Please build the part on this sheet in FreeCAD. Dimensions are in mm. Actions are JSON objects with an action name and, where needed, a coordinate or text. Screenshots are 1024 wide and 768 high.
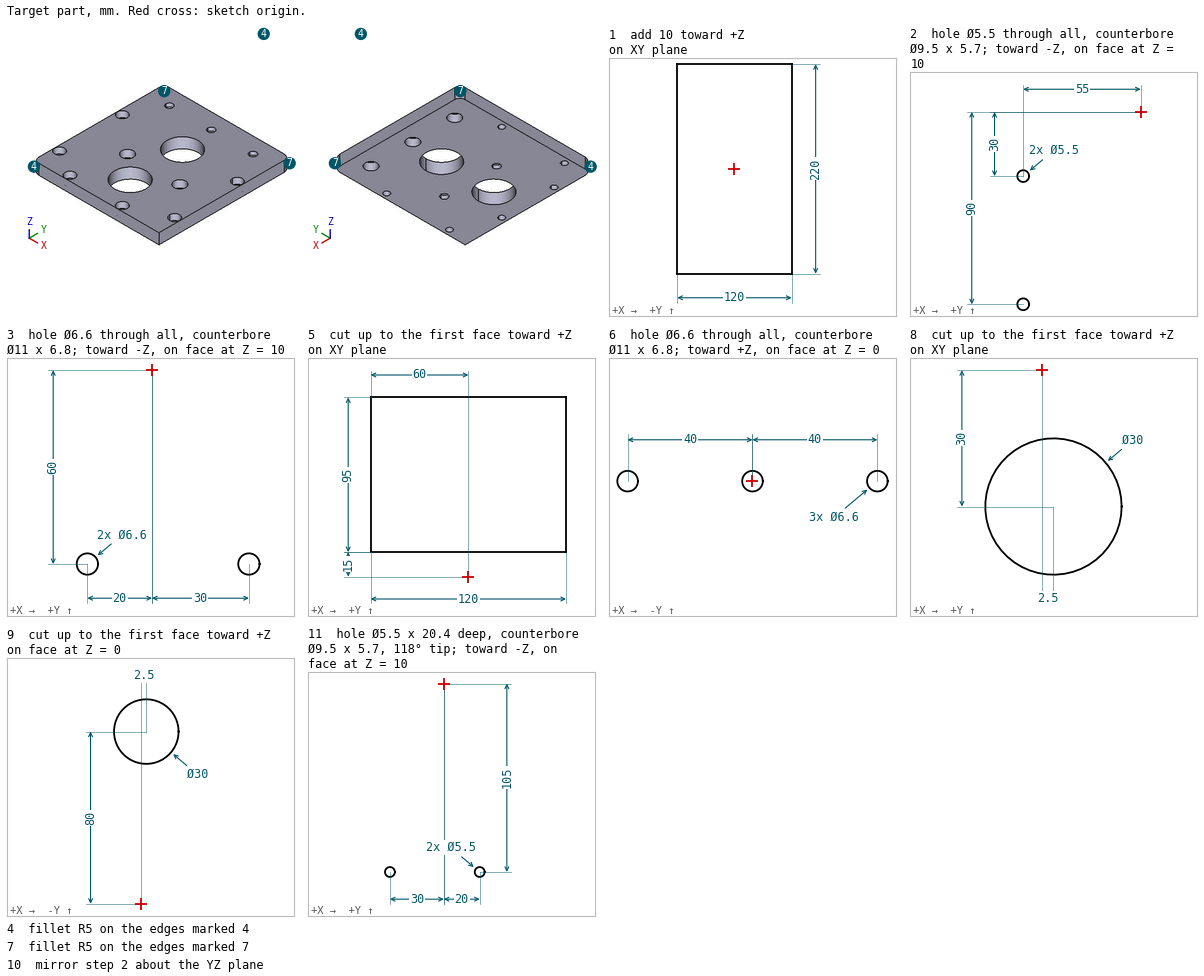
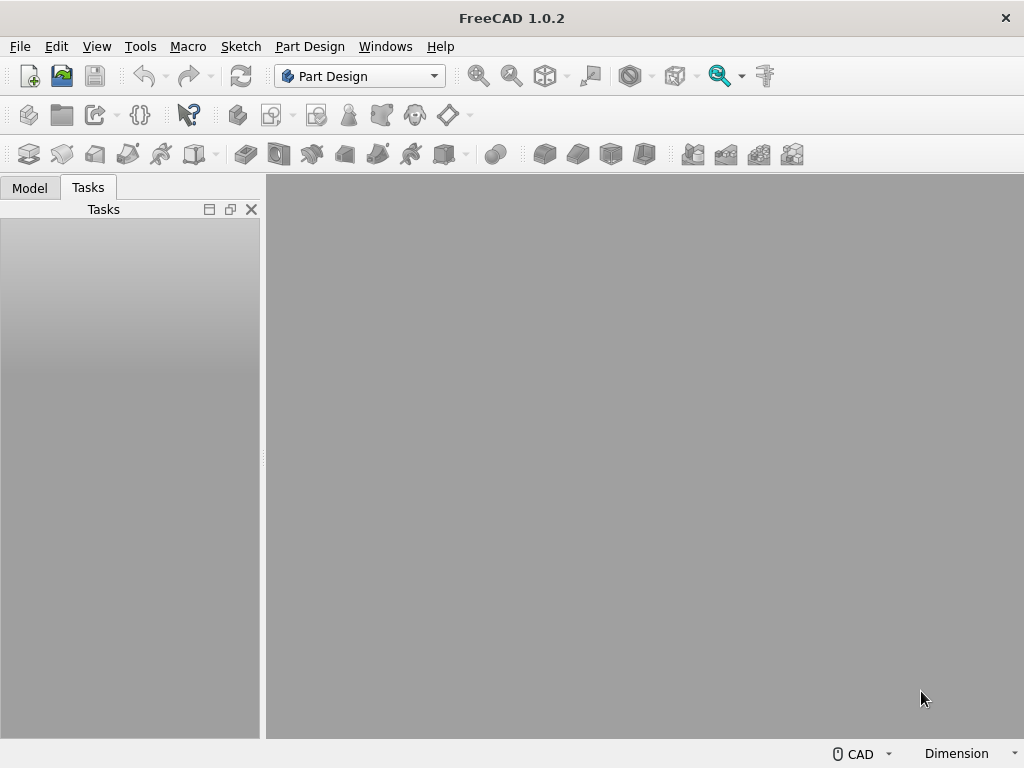
{"action": "left_click", "coordinate": [29, 76]}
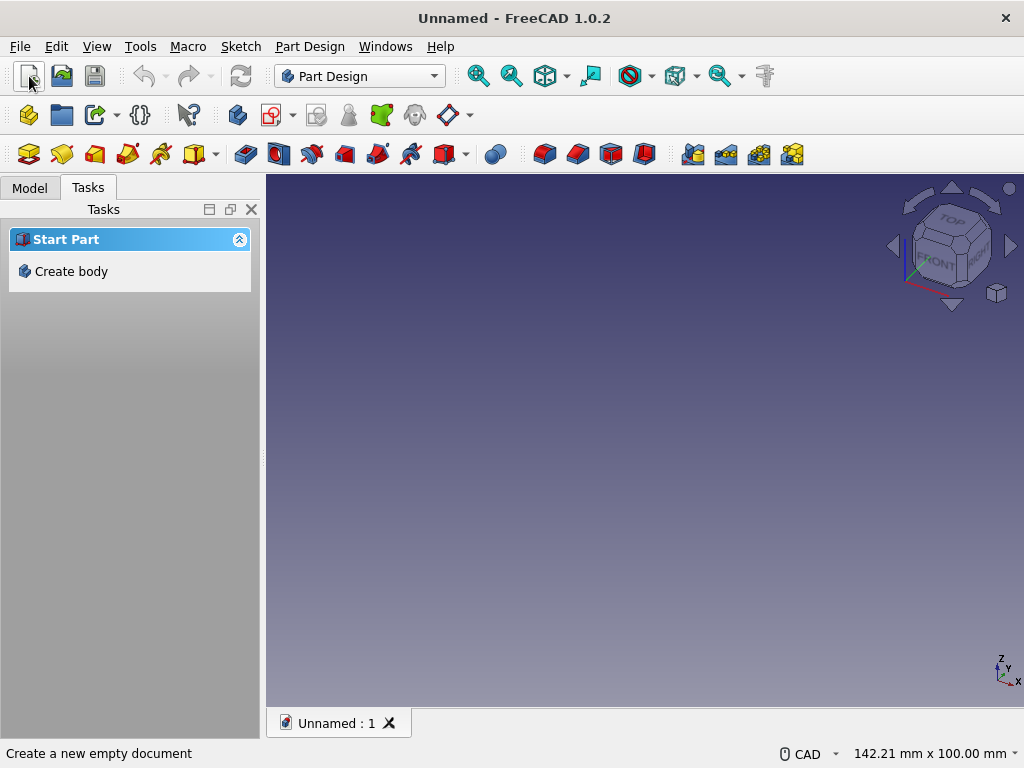
{"action": "left_click", "coordinate": [270, 116]}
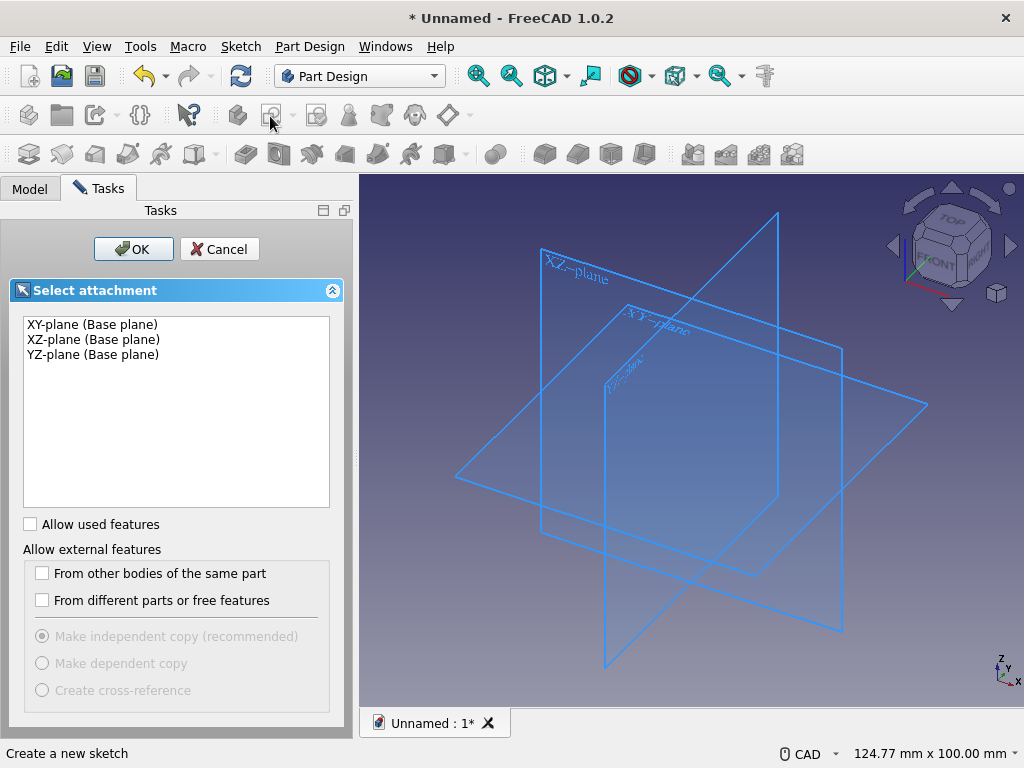
{"action": "left_click", "coordinate": [84, 324]}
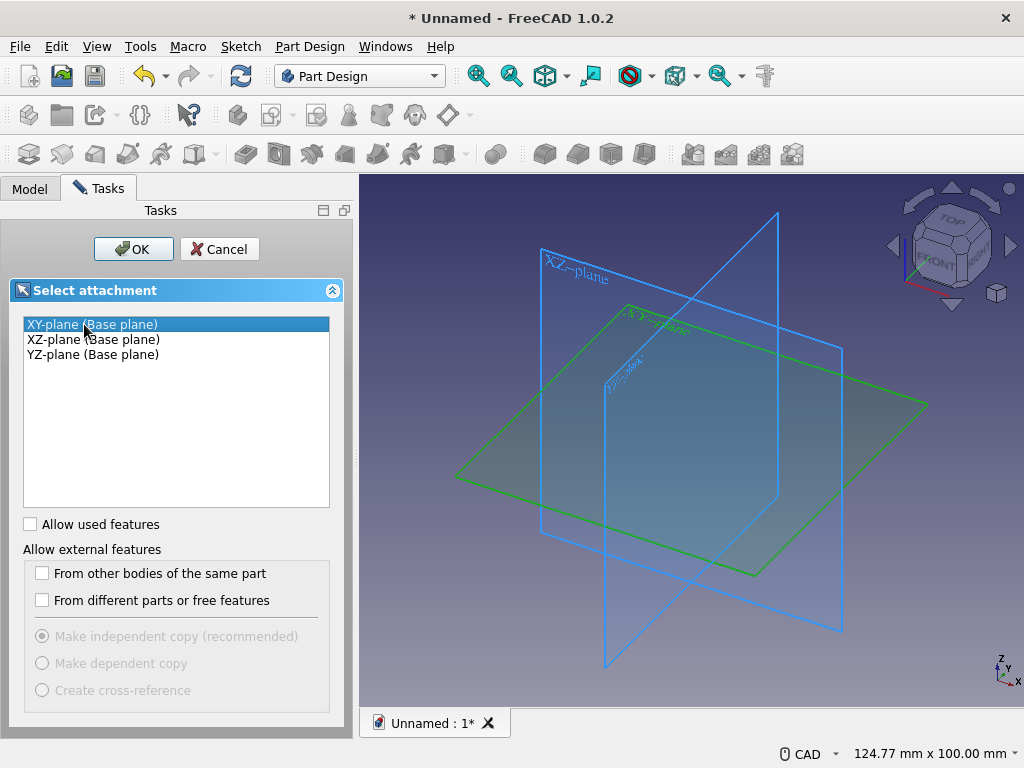
{"action": "left_click", "coordinate": [134, 249]}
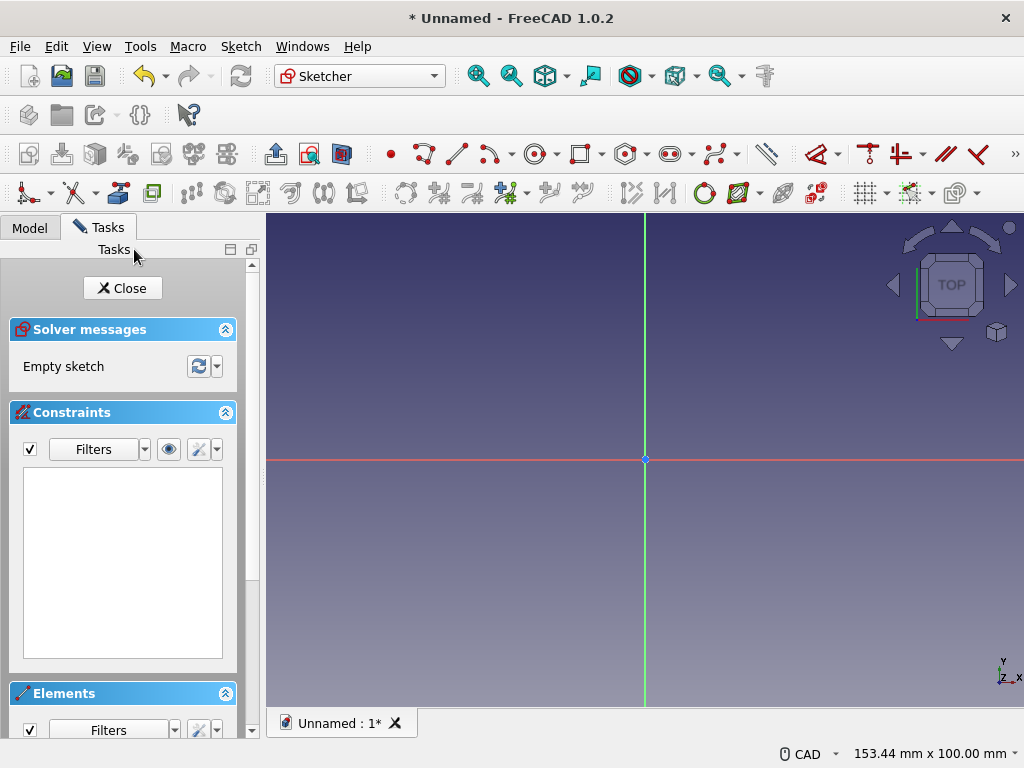
{"action": "scroll", "coordinate": [547, 460], "scroll_direction": "down", "scroll_amount": 6}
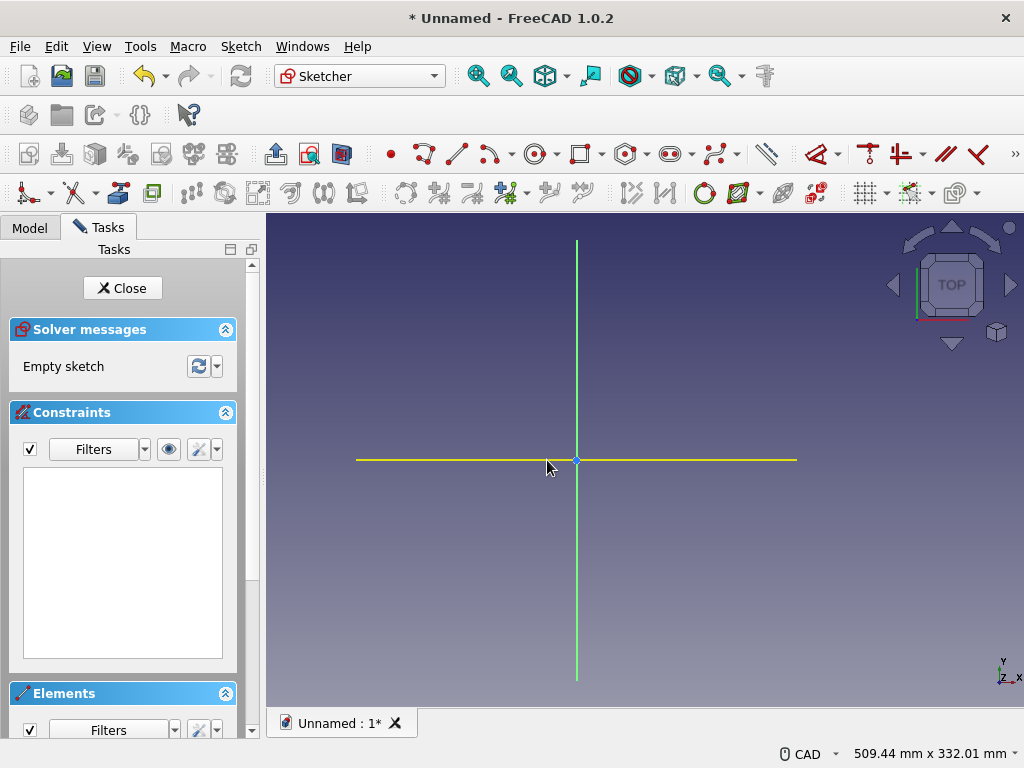
{"action": "left_click", "coordinate": [602, 154]}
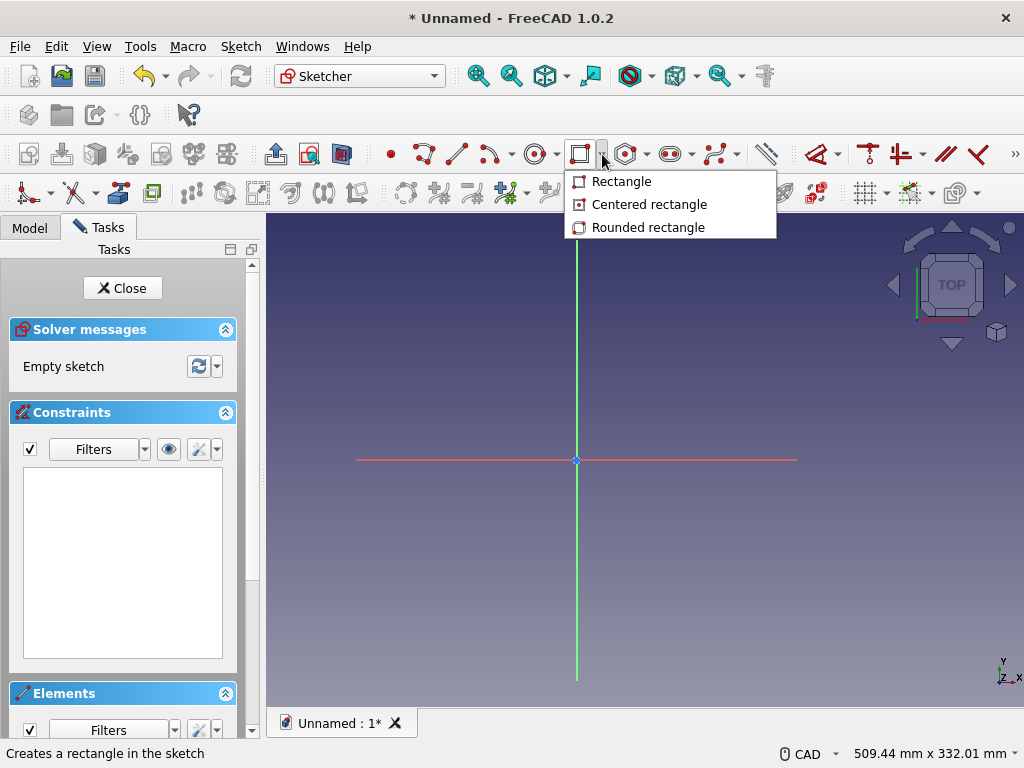
{"action": "left_click", "coordinate": [670, 204]}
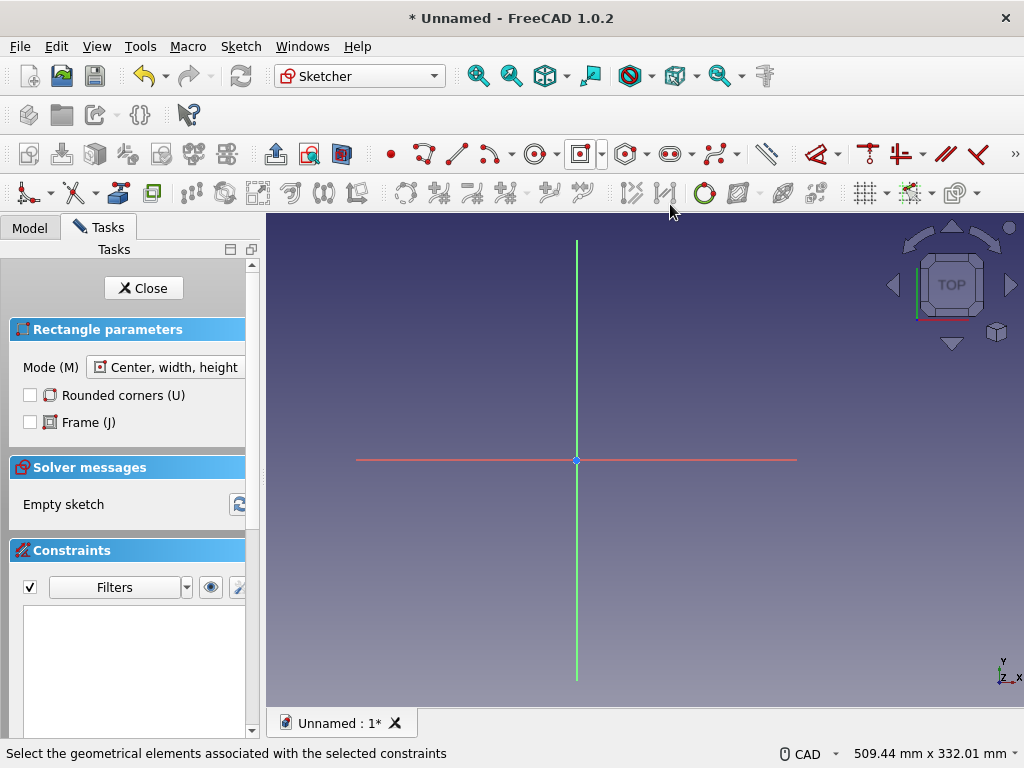
{"action": "left_click", "coordinate": [577, 460]}
{"action": "left_click", "coordinate": [666, 297]}
{"action": "key", "text": "Escape"}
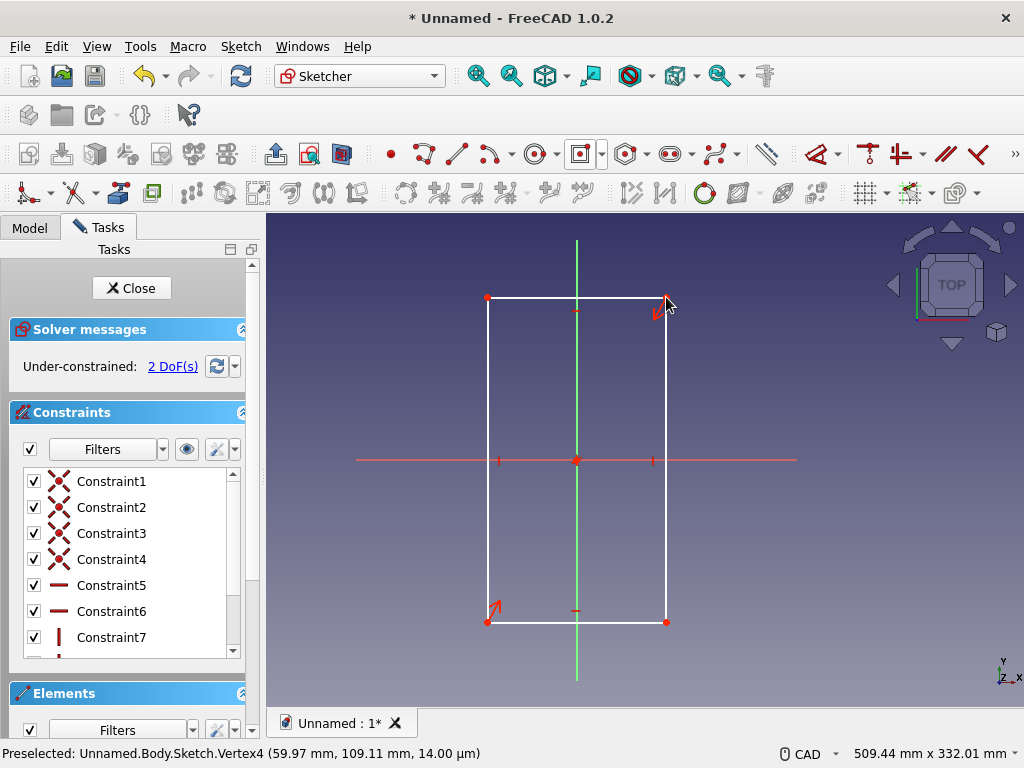
{"action": "left_click", "coordinate": [816, 154]}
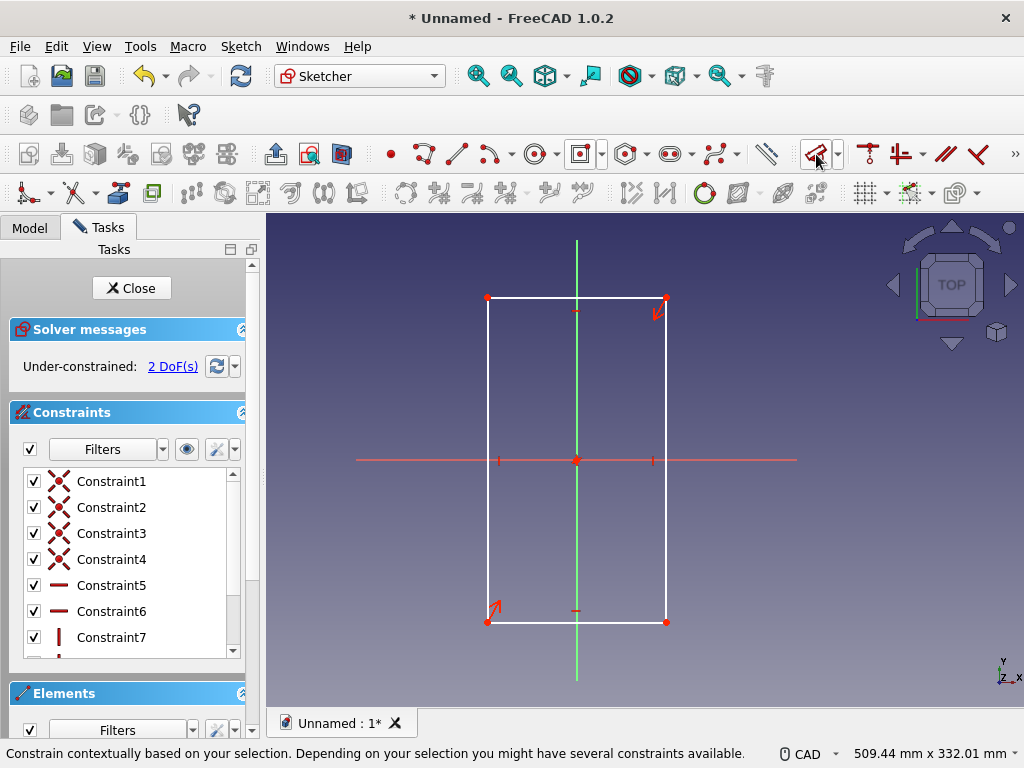
{"action": "left_click", "coordinate": [541, 623]}
{"action": "left_click", "coordinate": [536, 657]}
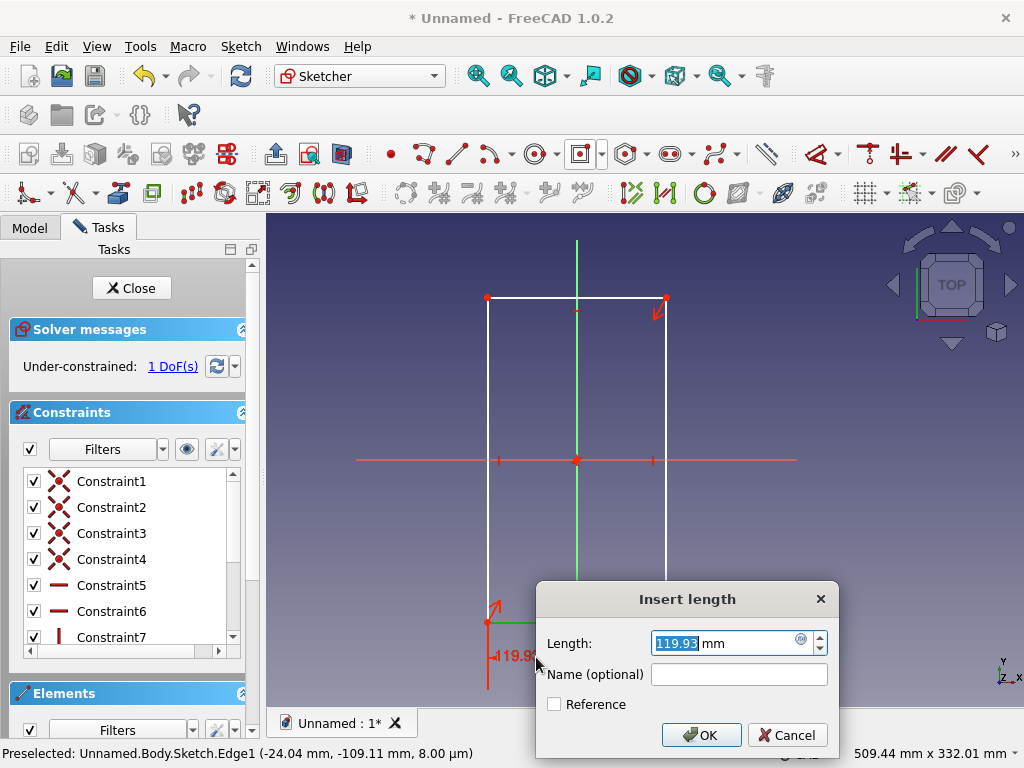
{"action": "type", "text": "120"}
{"action": "key", "text": "Return"}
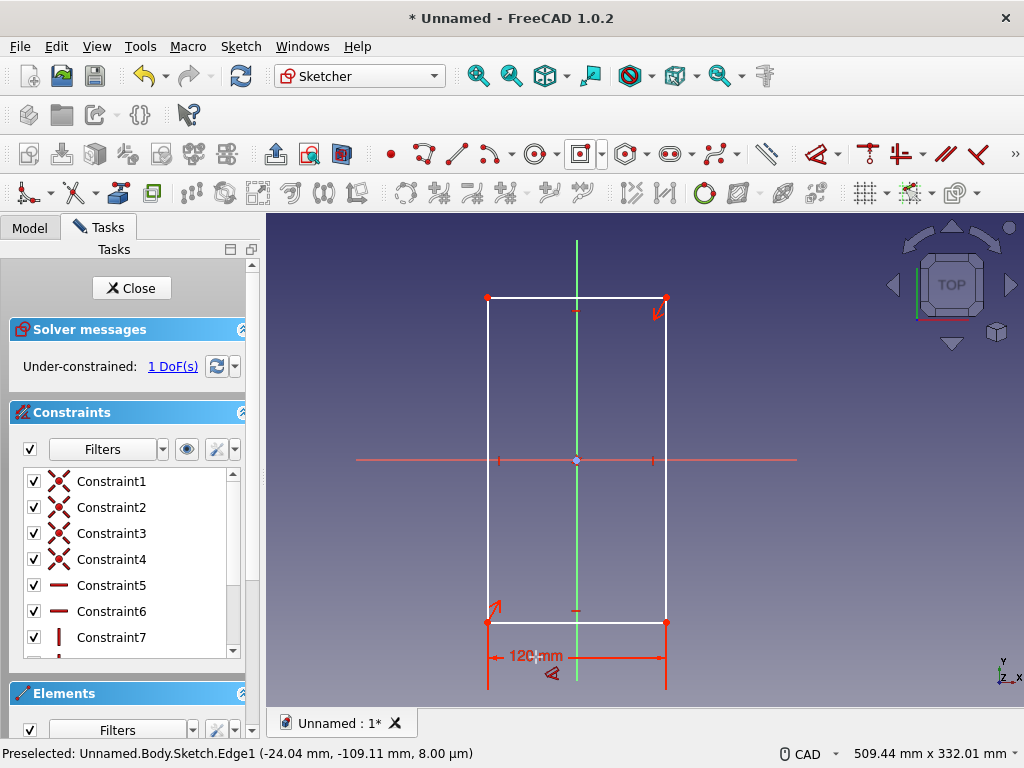
{"action": "left_click", "coordinate": [666, 525]}
{"action": "left_click", "coordinate": [700, 386]}